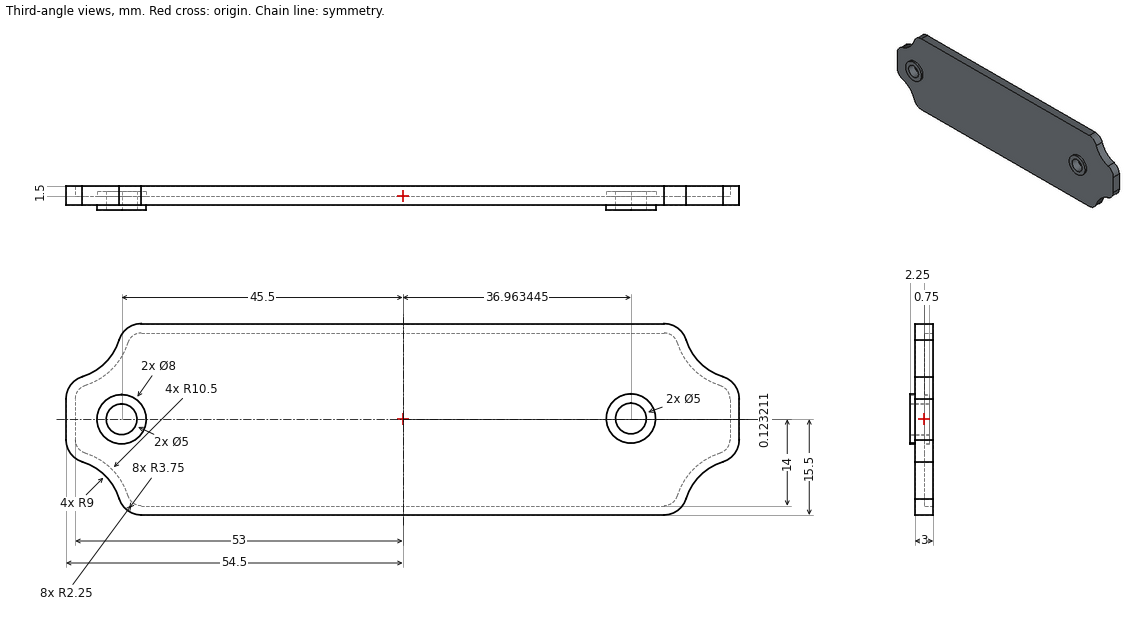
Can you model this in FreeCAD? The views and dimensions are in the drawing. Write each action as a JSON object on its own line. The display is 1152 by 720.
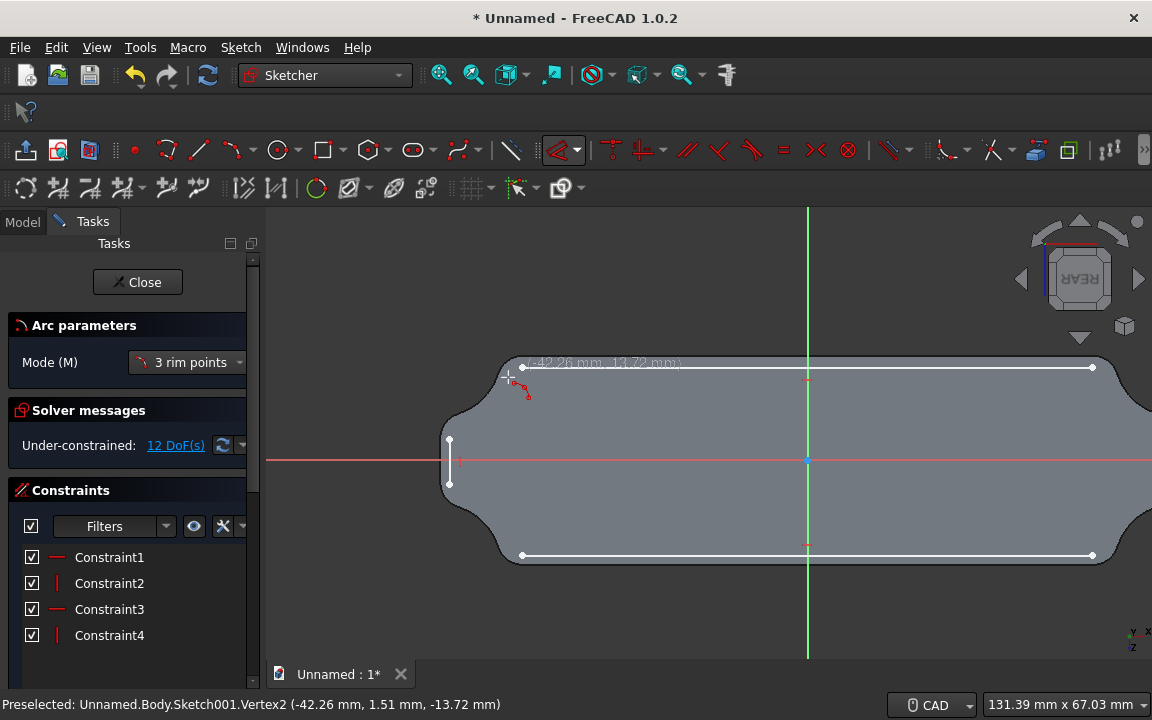
{"action": "left_click", "coordinate": [508, 377]}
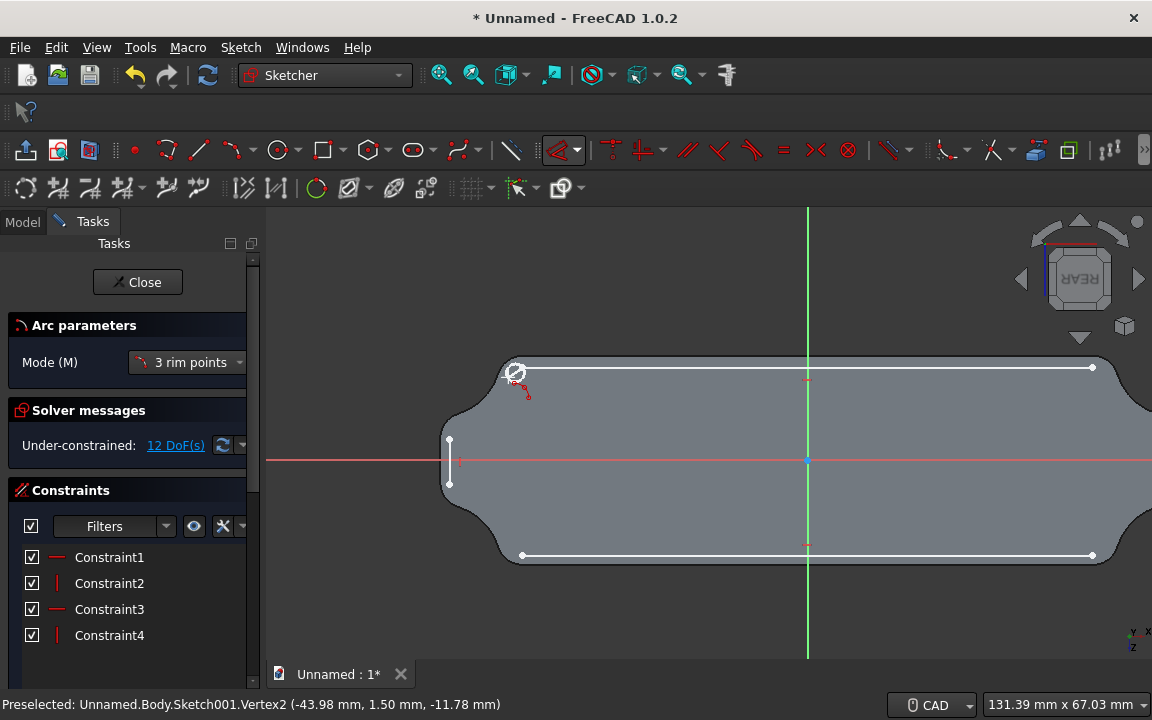
{"action": "scroll", "coordinate": [513, 369], "scroll_direction": "up", "scroll_amount": 9}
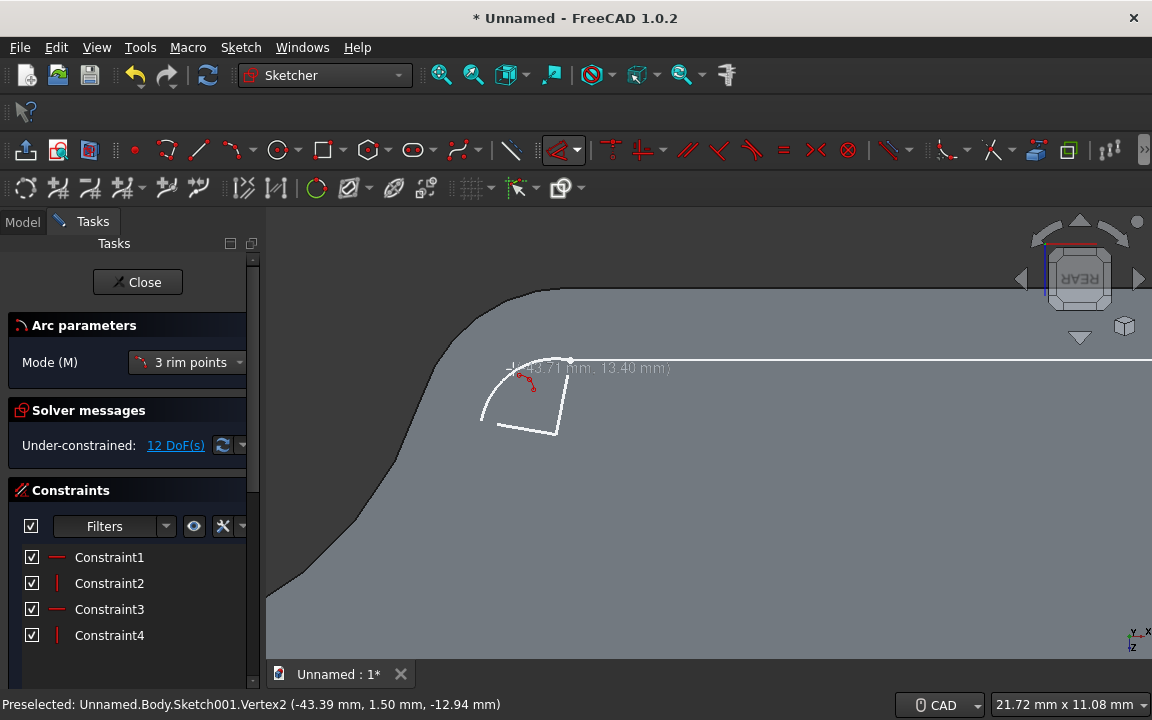
{"action": "left_click", "coordinate": [514, 367]}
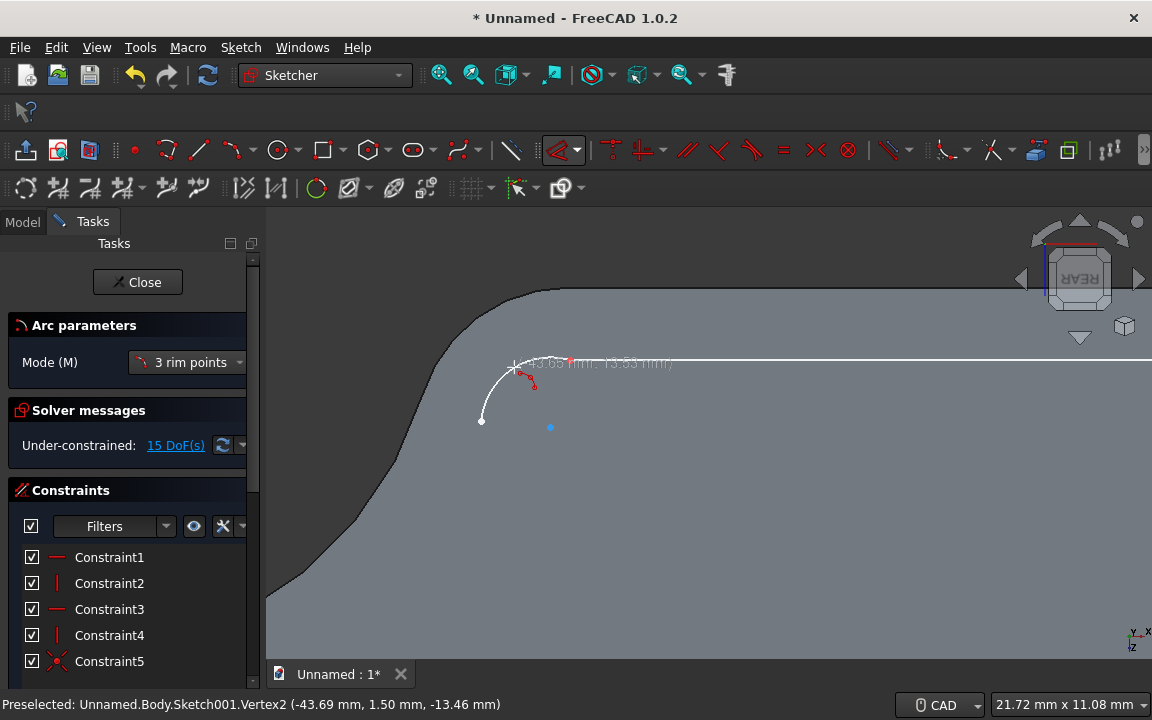
{"action": "scroll", "coordinate": [434, 372], "scroll_direction": "down", "scroll_amount": 11}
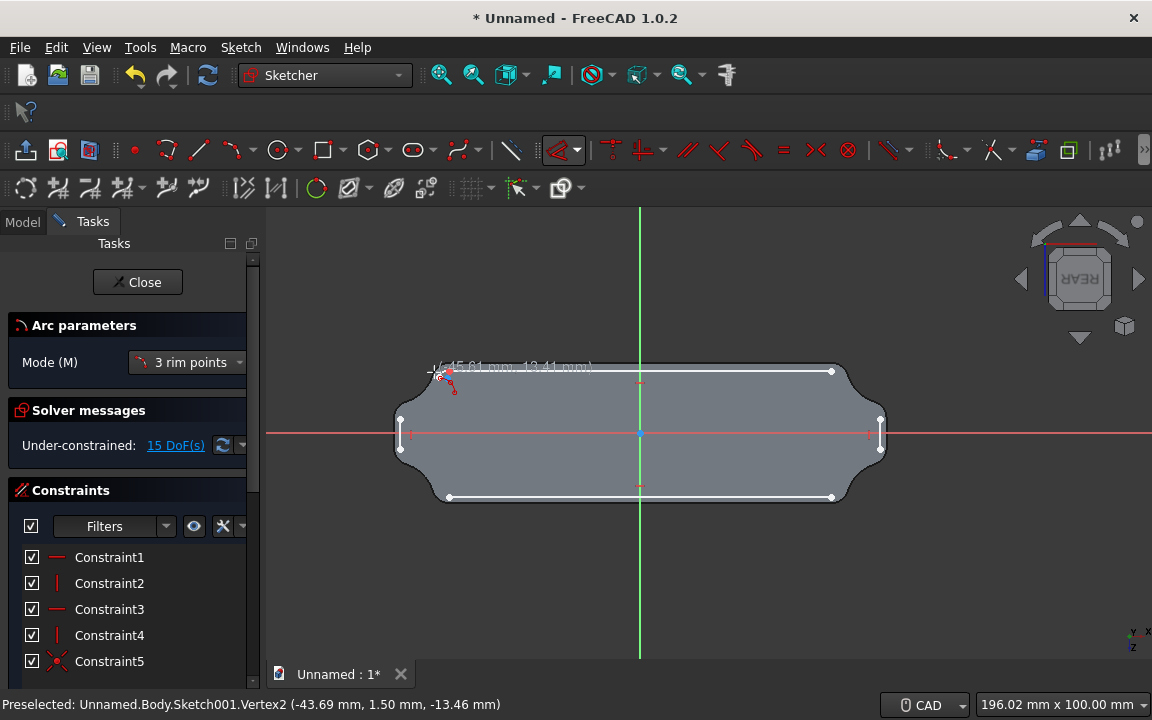
{"action": "scroll", "coordinate": [439, 377], "scroll_direction": "up", "scroll_amount": 3}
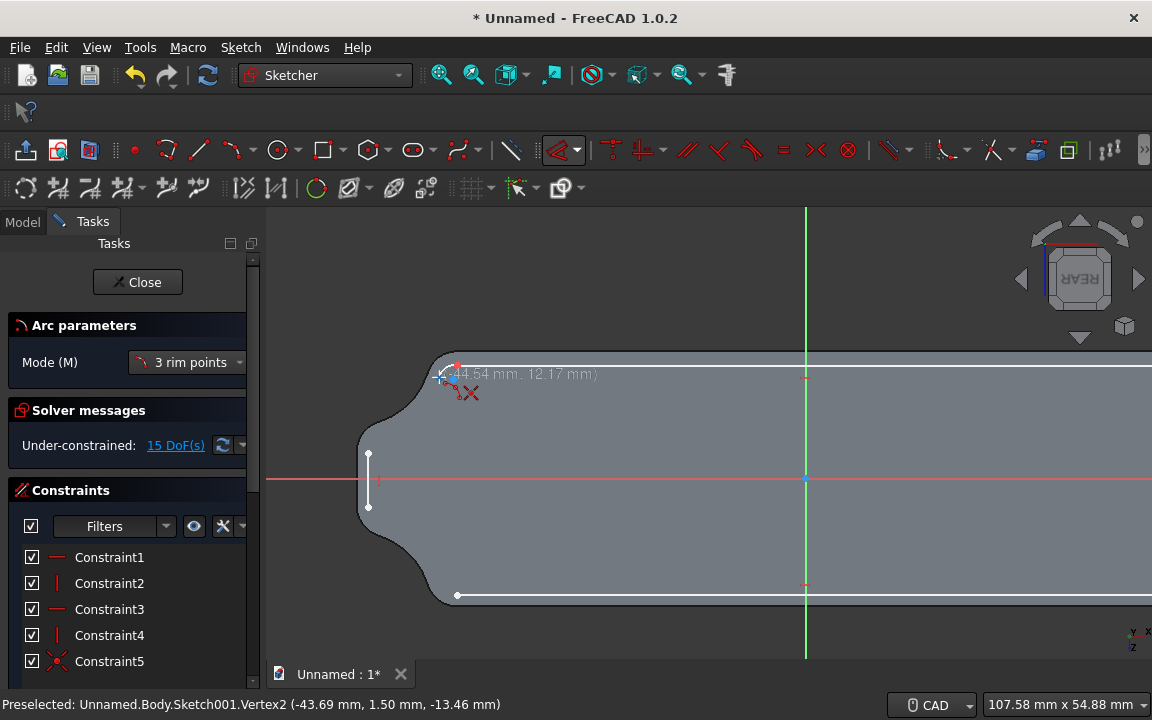
{"action": "left_click", "coordinate": [440, 378]}
{"action": "left_click", "coordinate": [382, 434]}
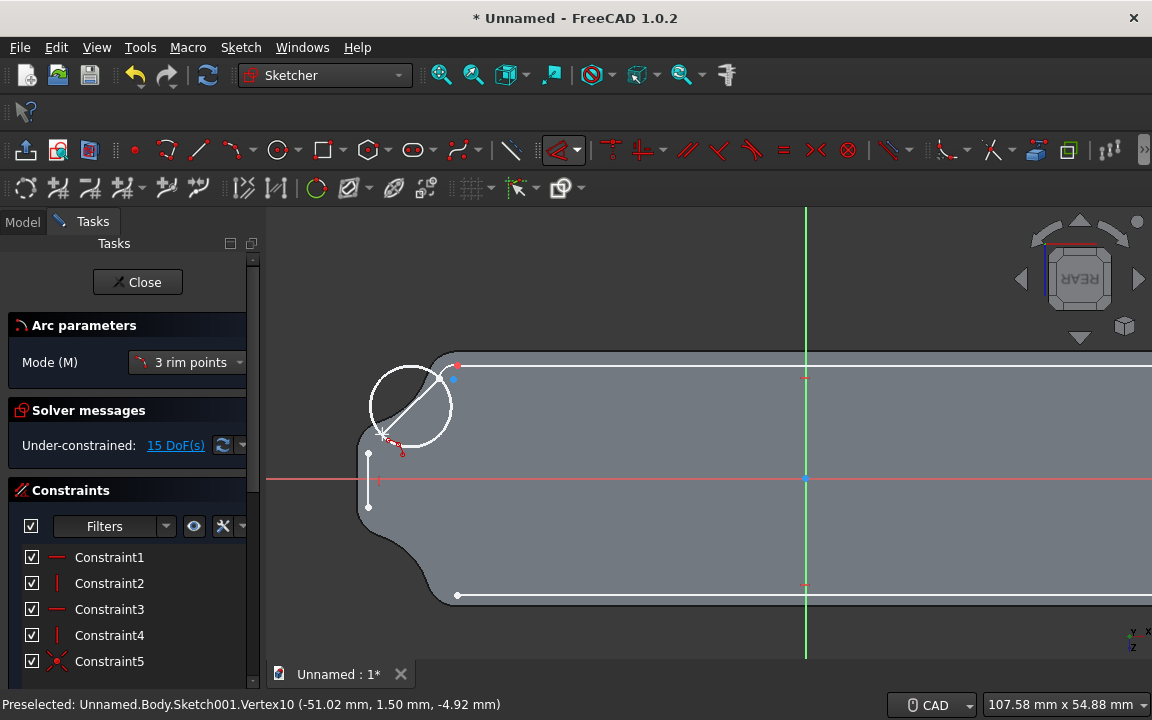
{"action": "scroll", "coordinate": [418, 412], "scroll_direction": "up", "scroll_amount": 3}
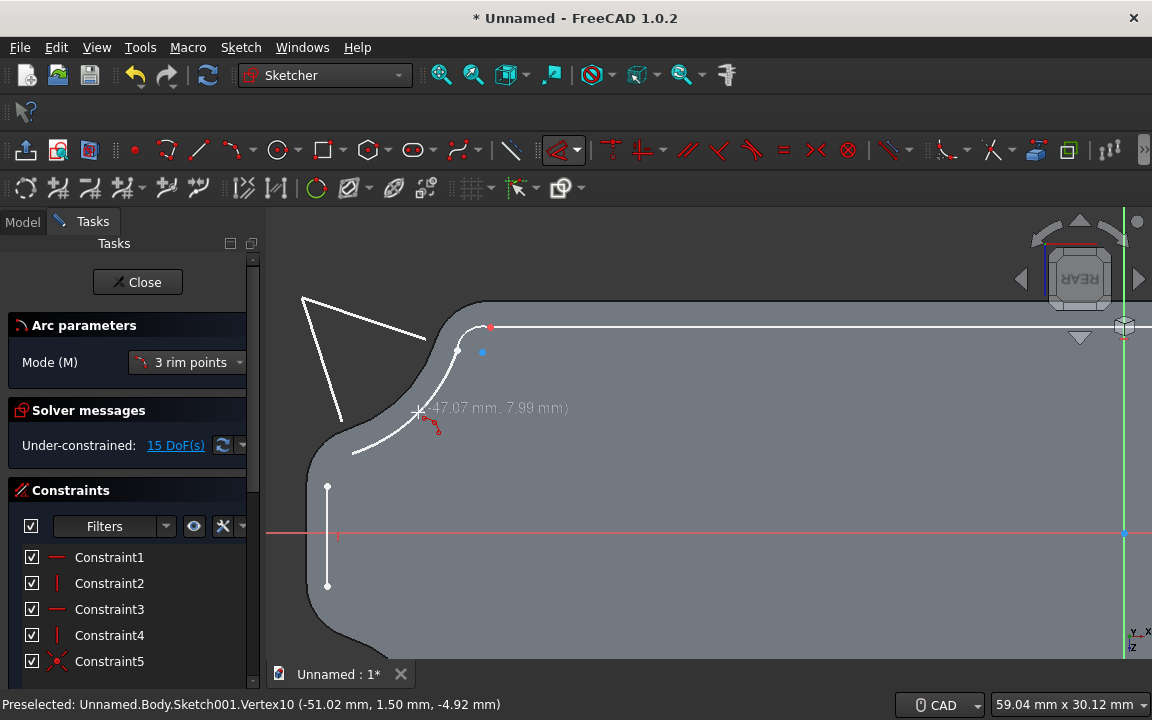
{"action": "left_click", "coordinate": [418, 412]}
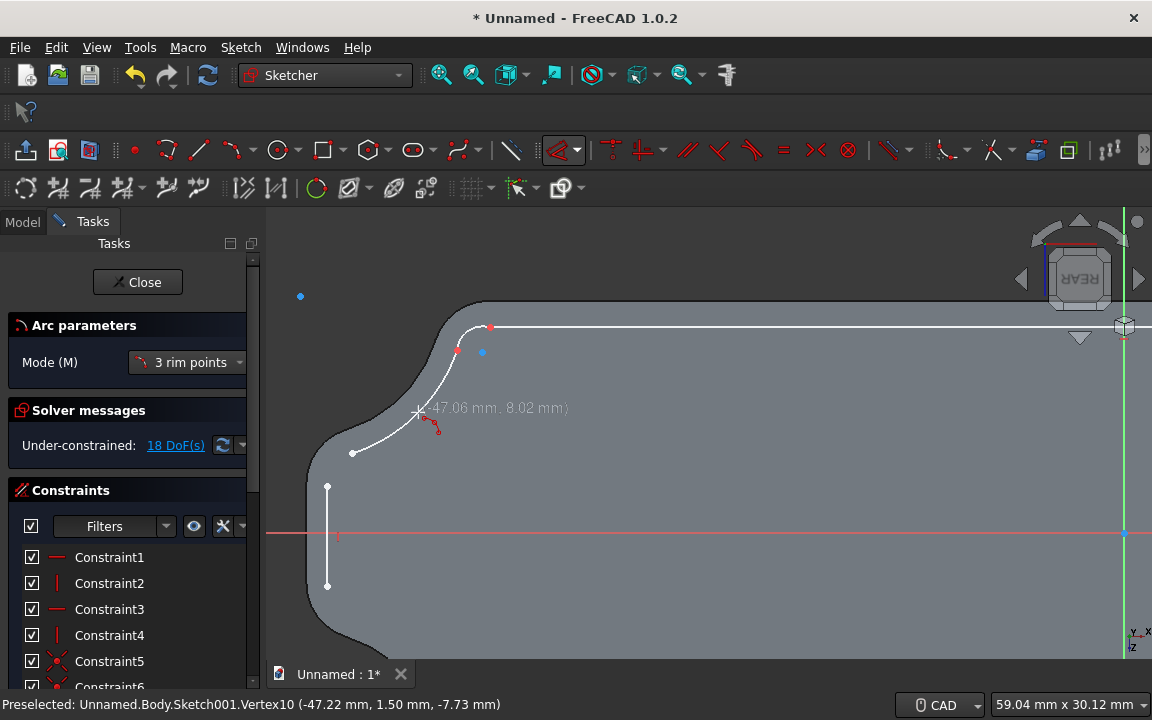
{"action": "left_click", "coordinate": [352, 454]}
{"action": "left_click", "coordinate": [327, 487]}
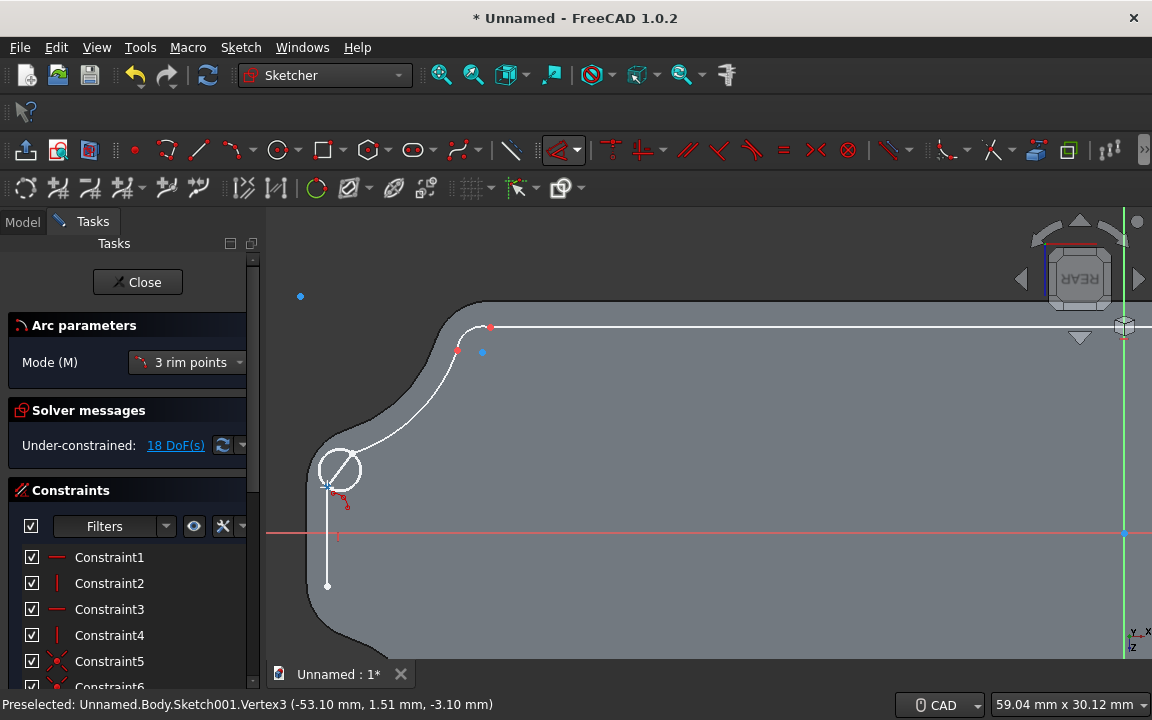
{"action": "scroll", "coordinate": [335, 464], "scroll_direction": "up", "scroll_amount": 5}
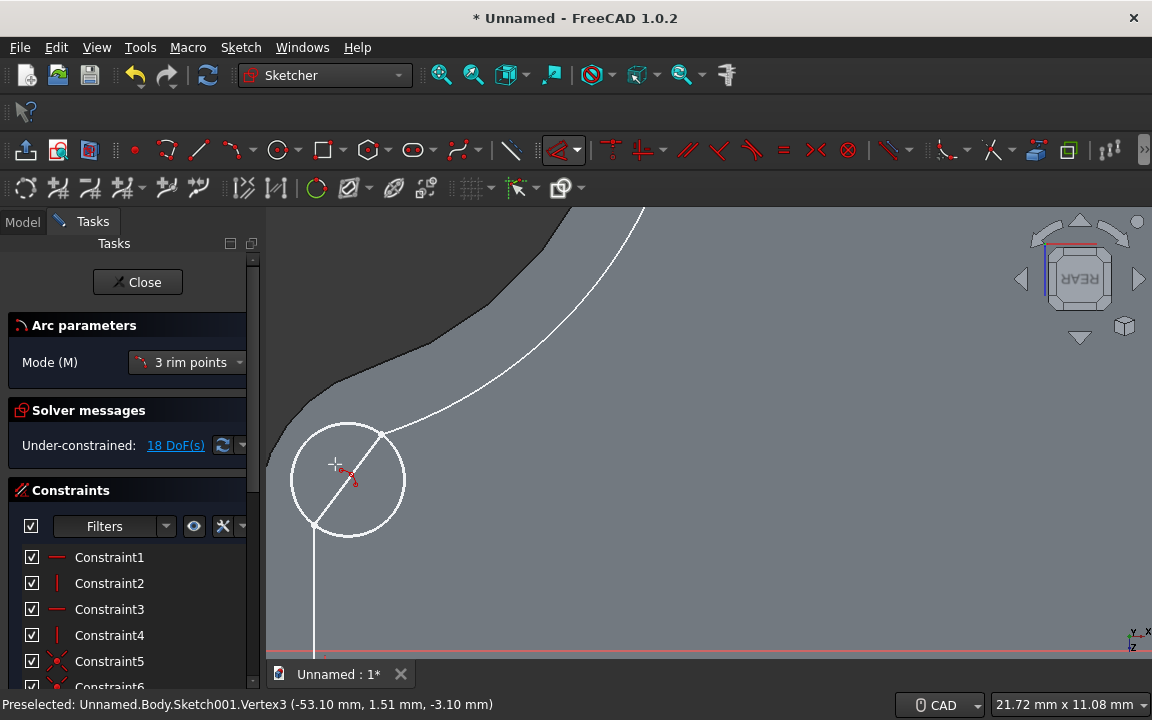
{"action": "left_click", "coordinate": [336, 462]}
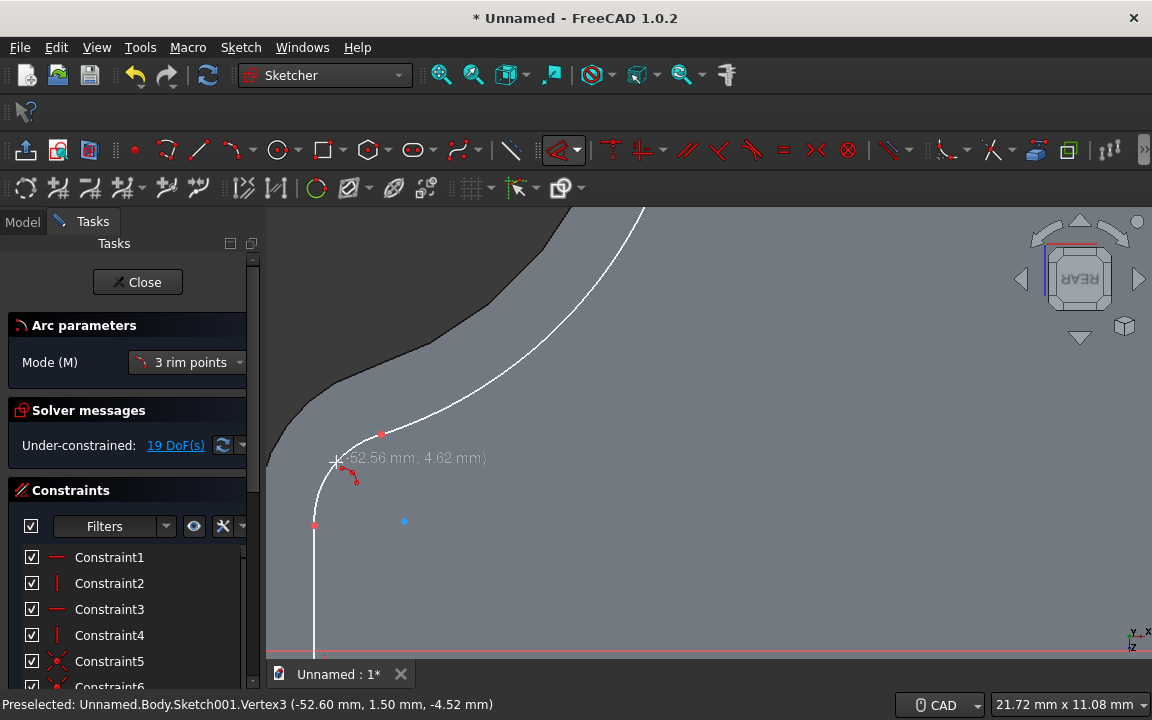
{"action": "scroll", "coordinate": [411, 406], "scroll_direction": "down", "scroll_amount": 11}